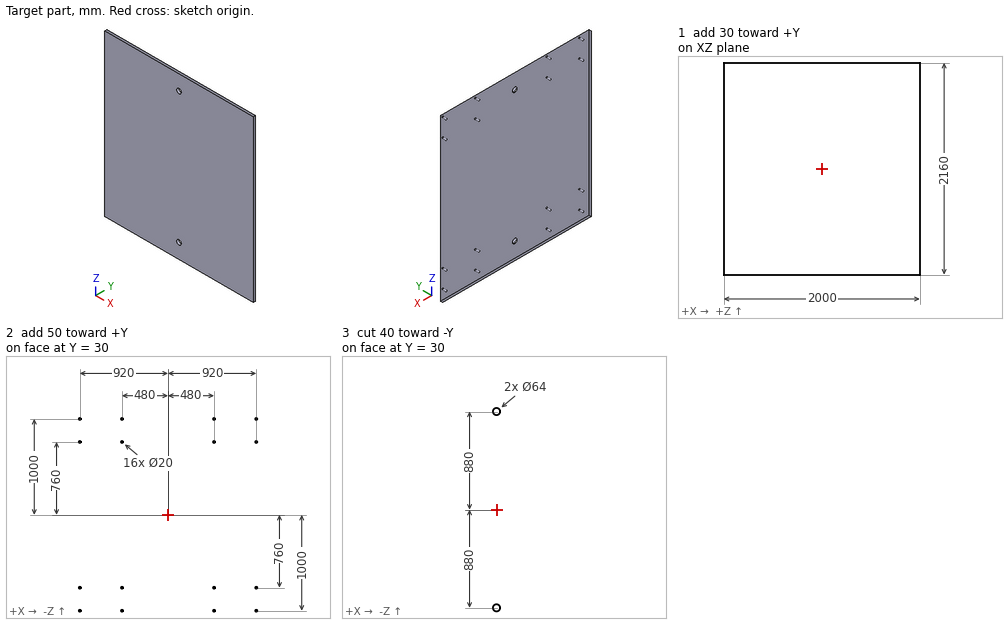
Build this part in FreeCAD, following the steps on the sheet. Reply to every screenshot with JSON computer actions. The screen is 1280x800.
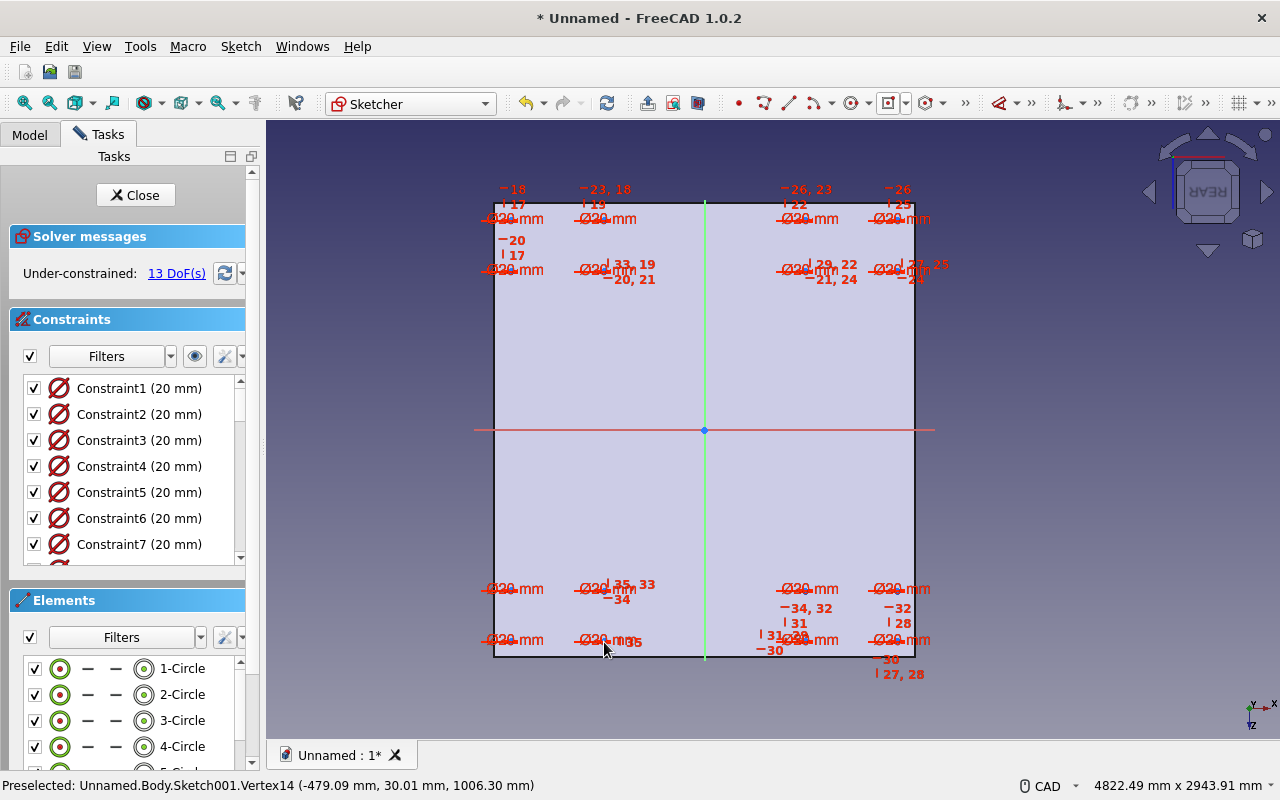
{"action": "left_click", "coordinate": [806, 642]}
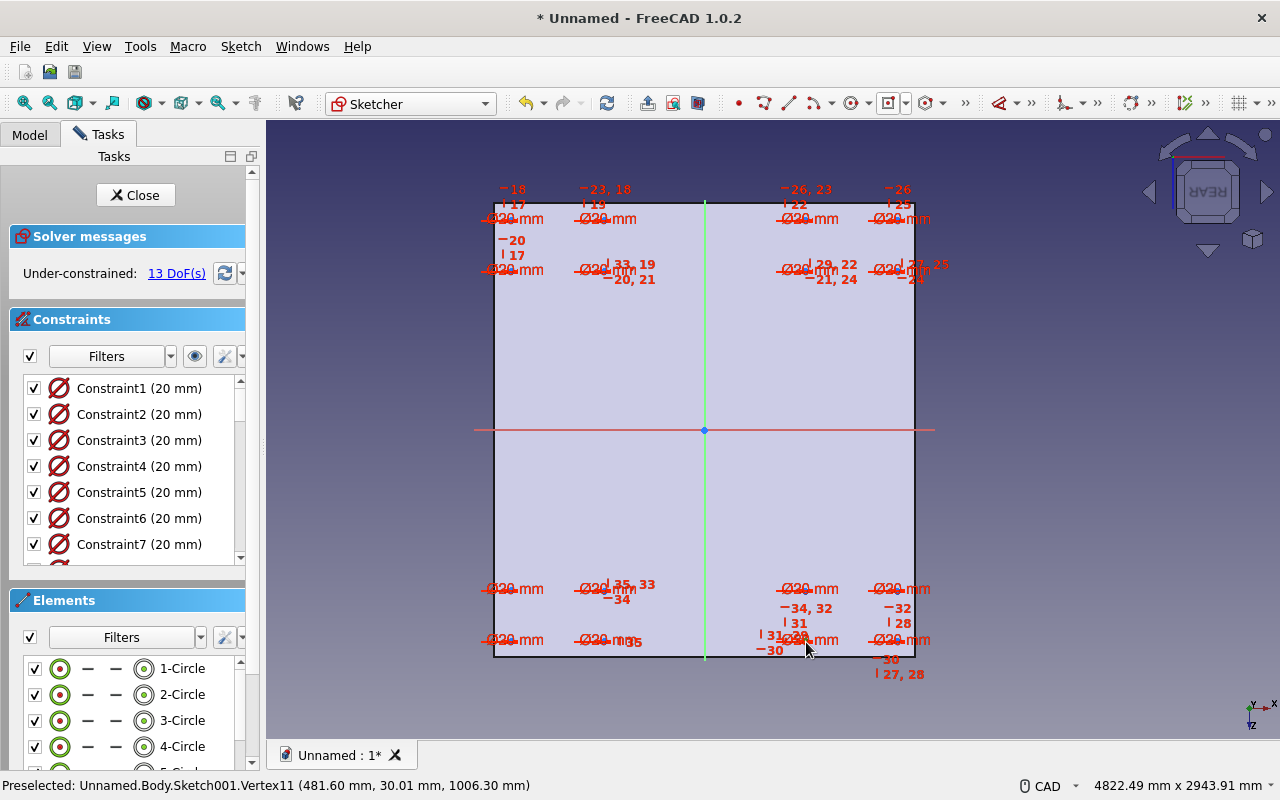
{"action": "left_click", "coordinate": [604, 642]}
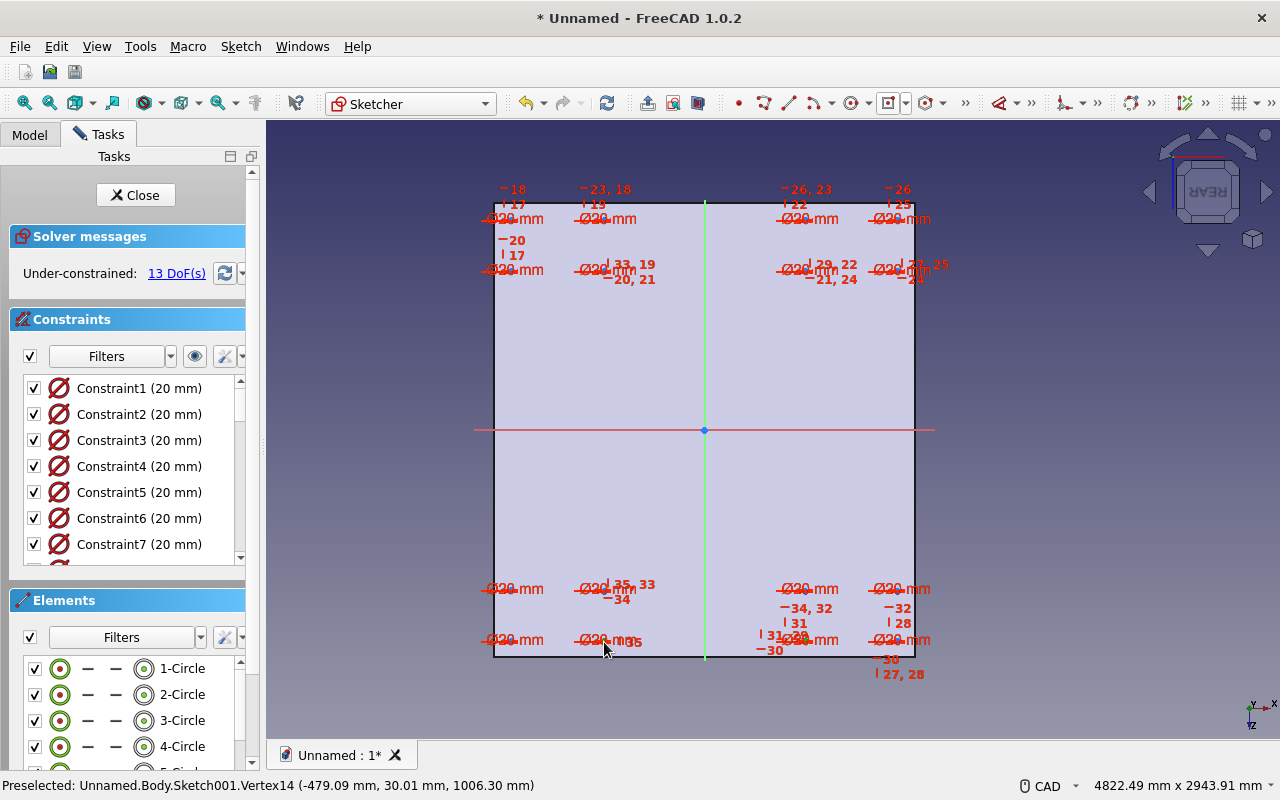
{"action": "key", "text": "h"}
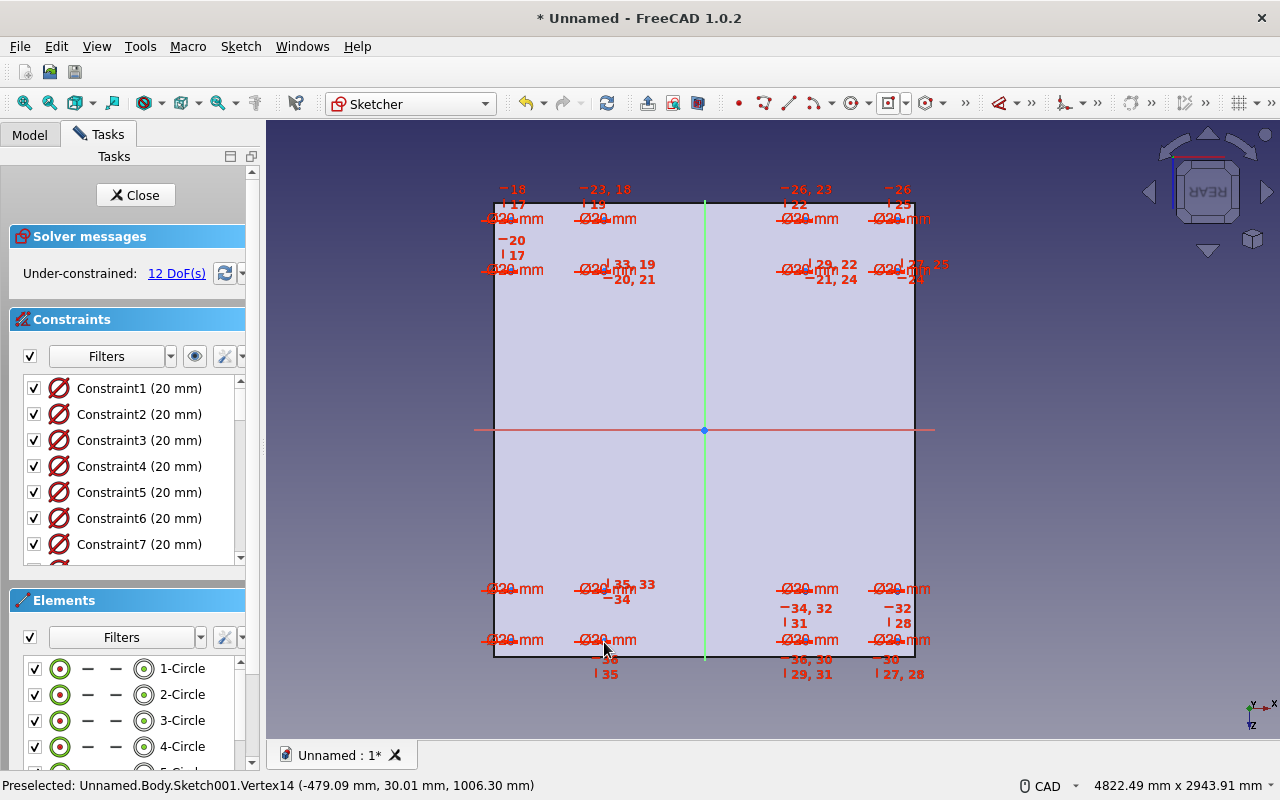
{"action": "left_click", "coordinate": [511, 272]}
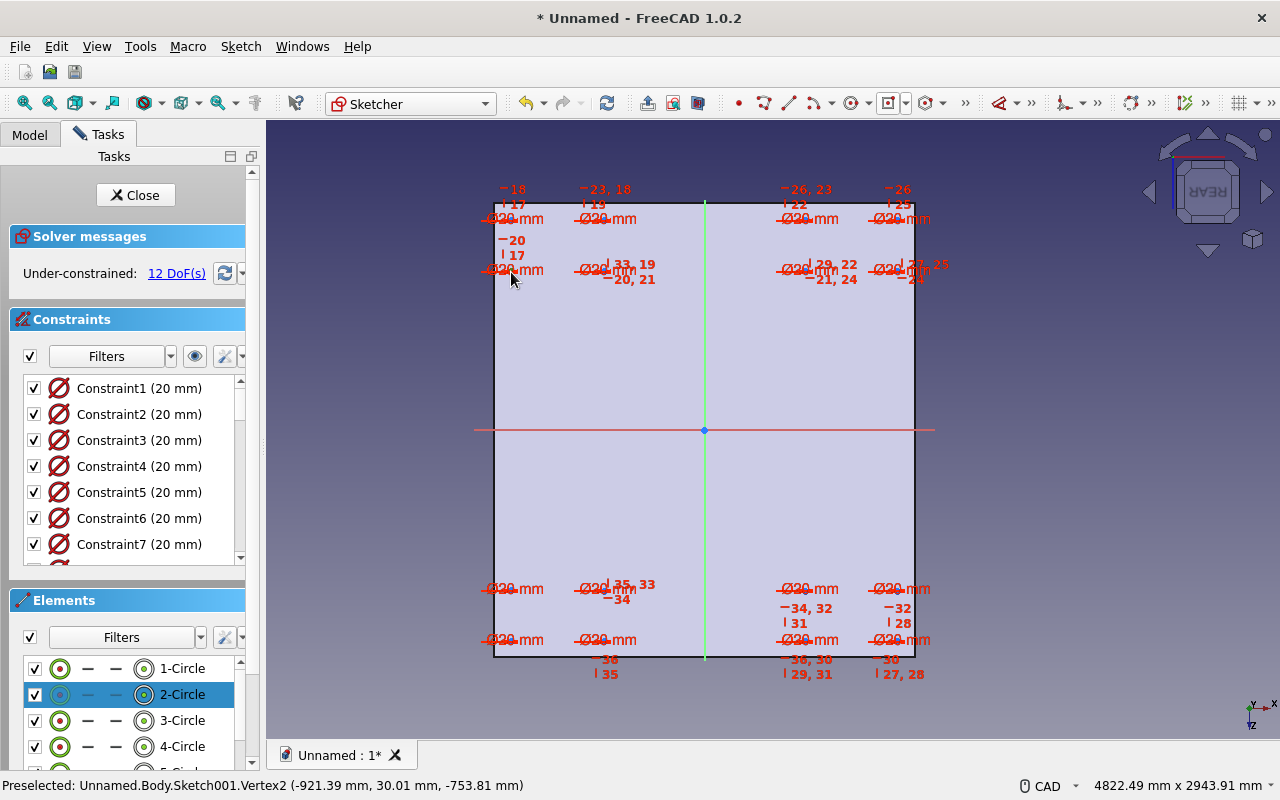
{"action": "left_click", "coordinate": [511, 591]}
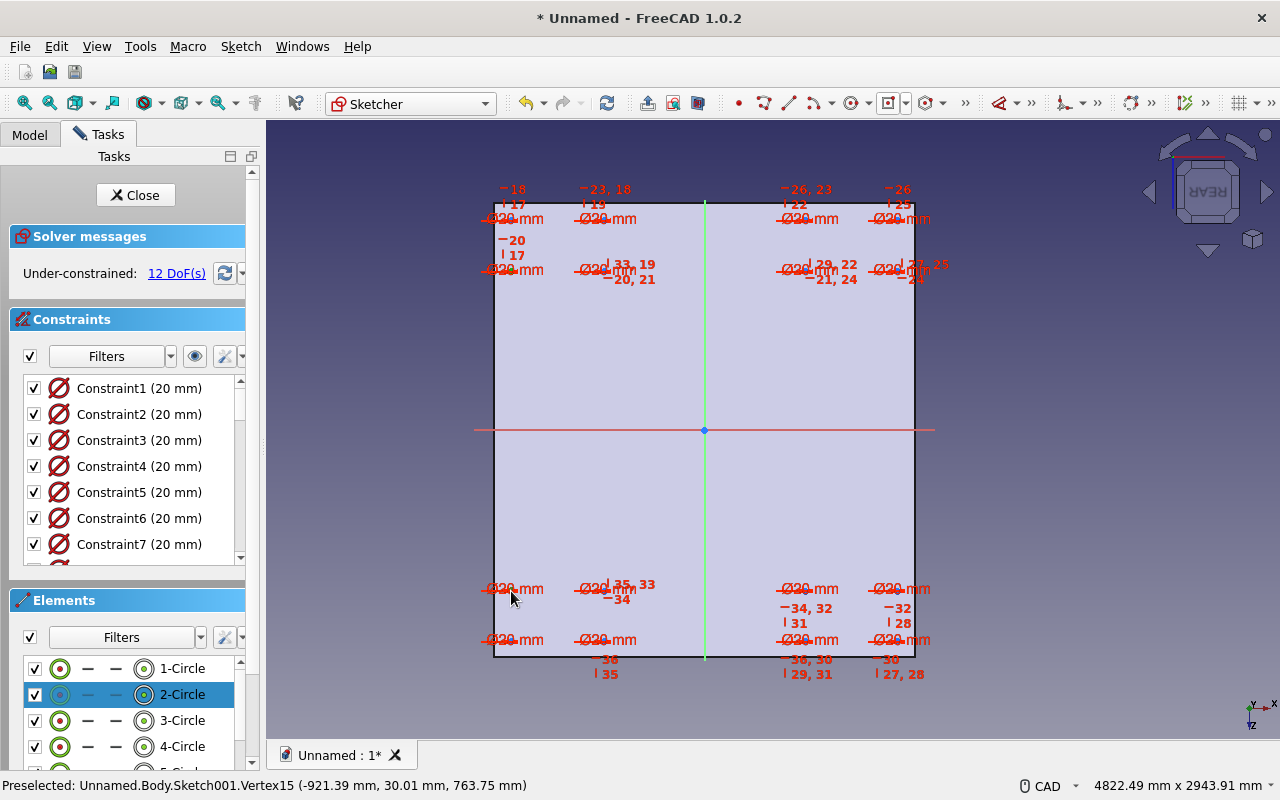
{"action": "key", "text": "v"}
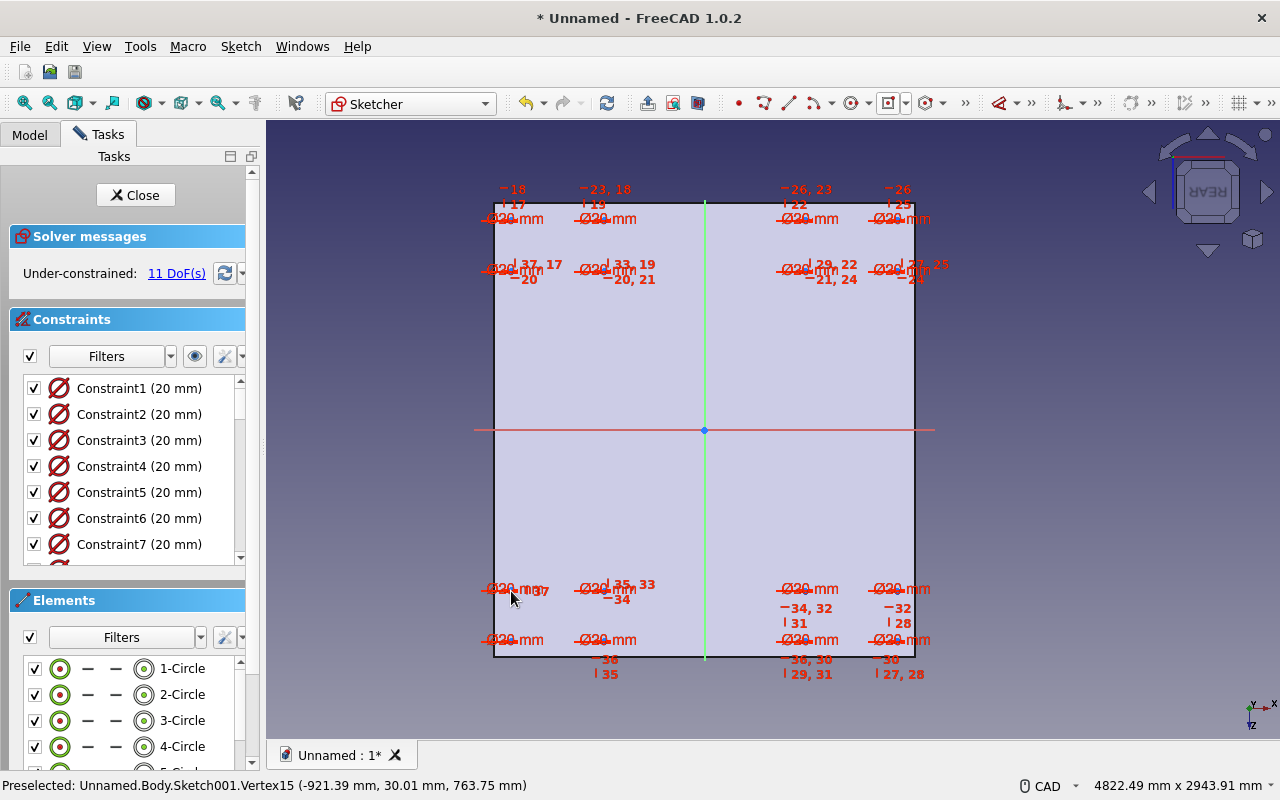
{"action": "left_click", "coordinate": [604, 591]}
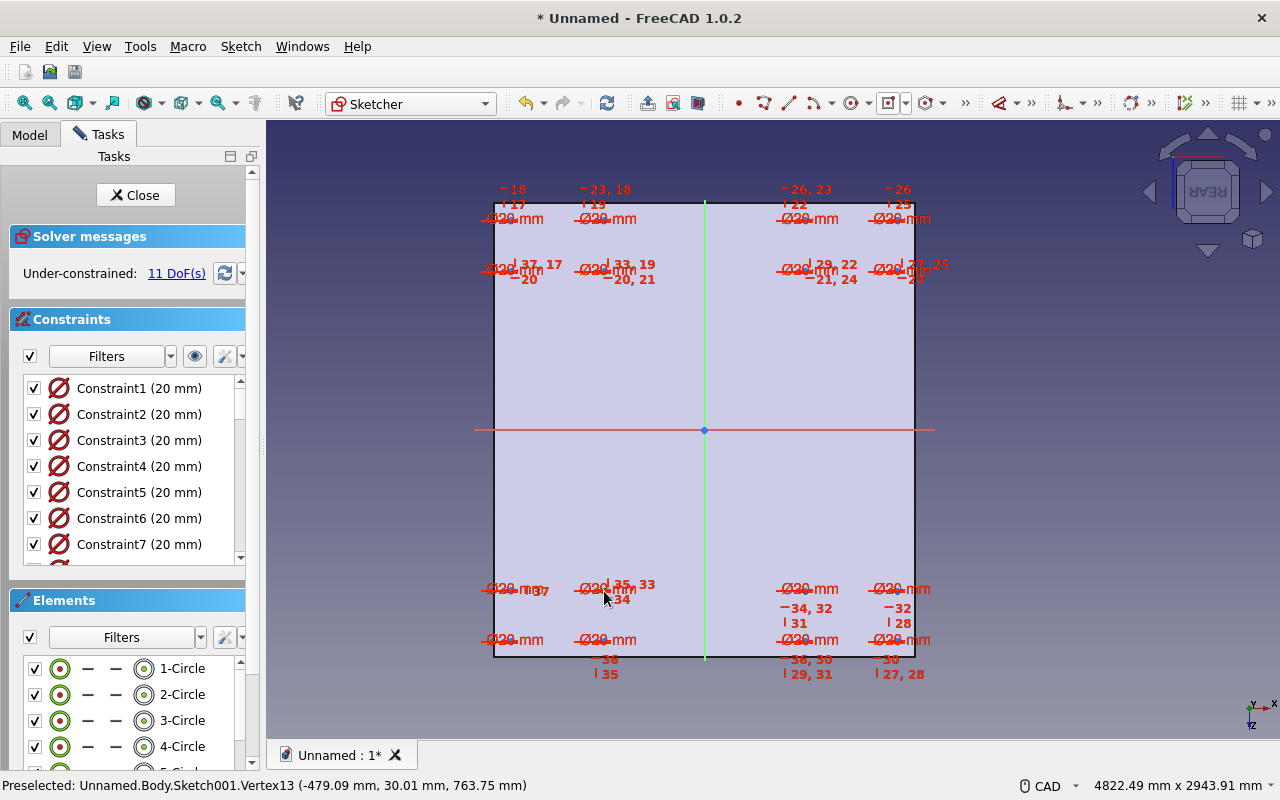
{"action": "left_click", "coordinate": [511, 591]}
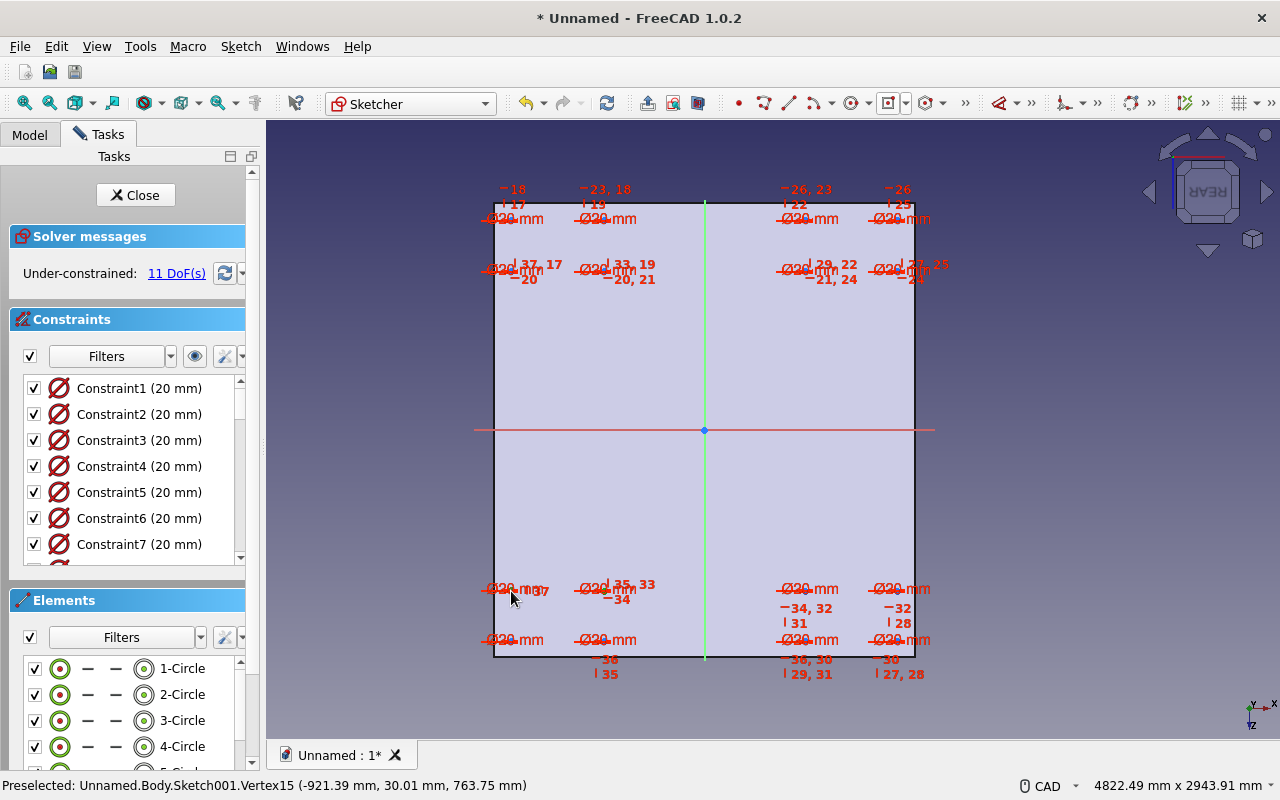
{"action": "key", "text": "h"}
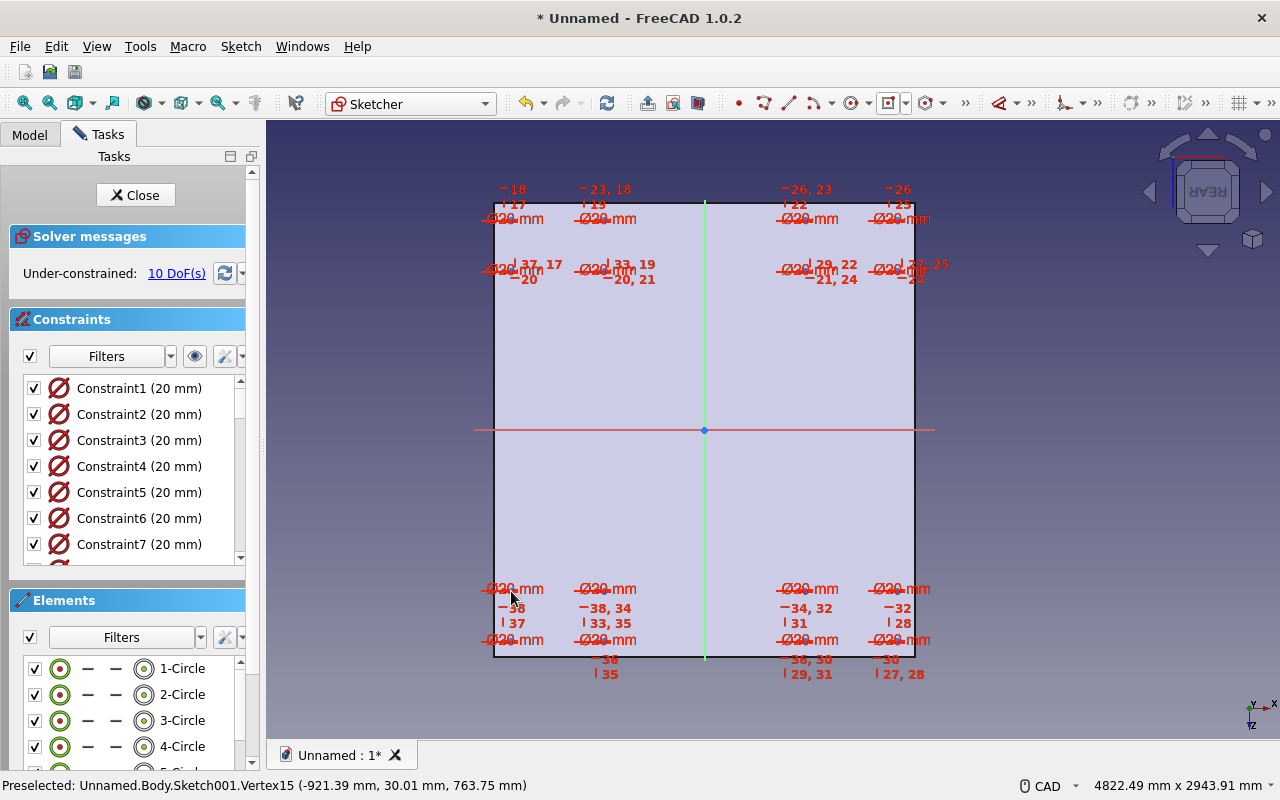
{"action": "left_click", "coordinate": [511, 591]}